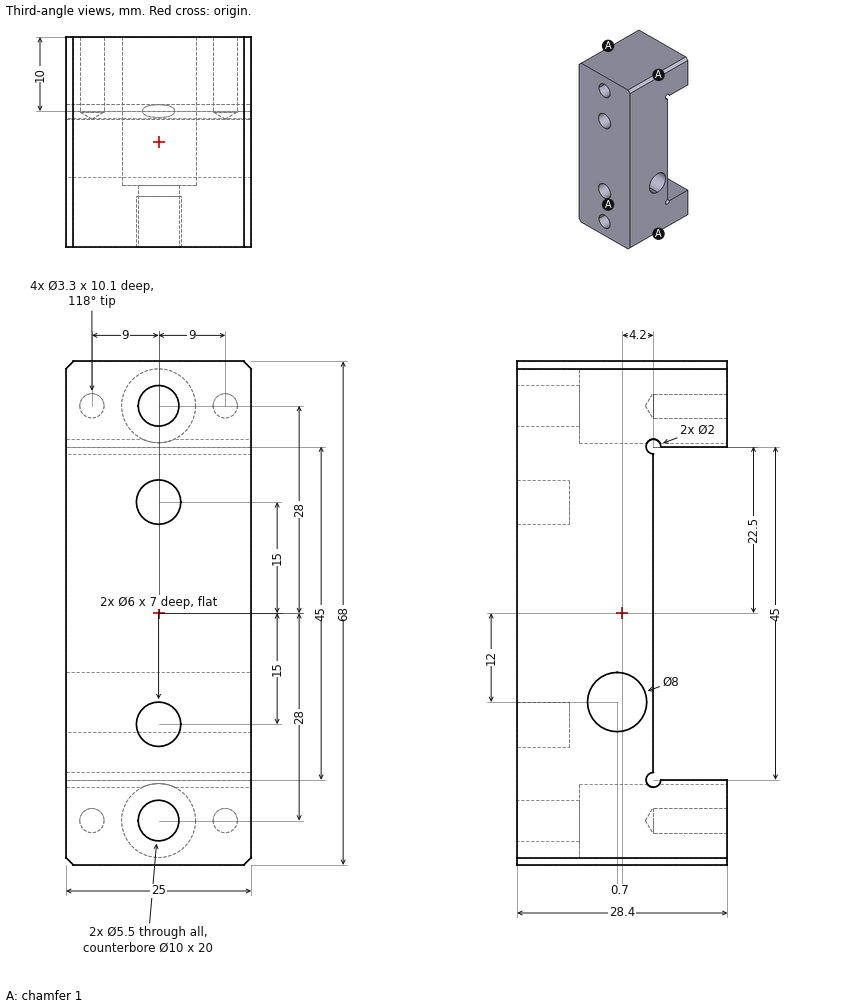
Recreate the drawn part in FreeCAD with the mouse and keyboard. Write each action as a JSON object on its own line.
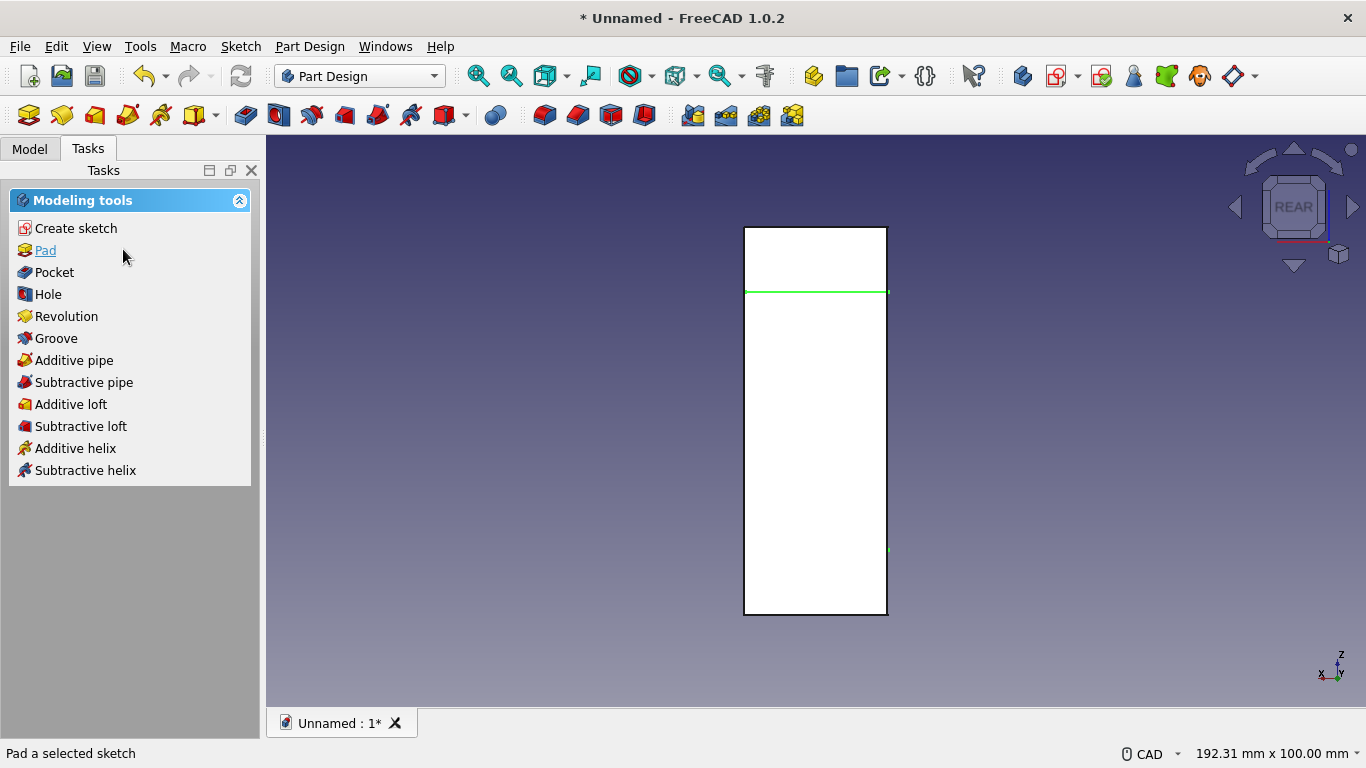
{"action": "left_click", "coordinate": [246, 116]}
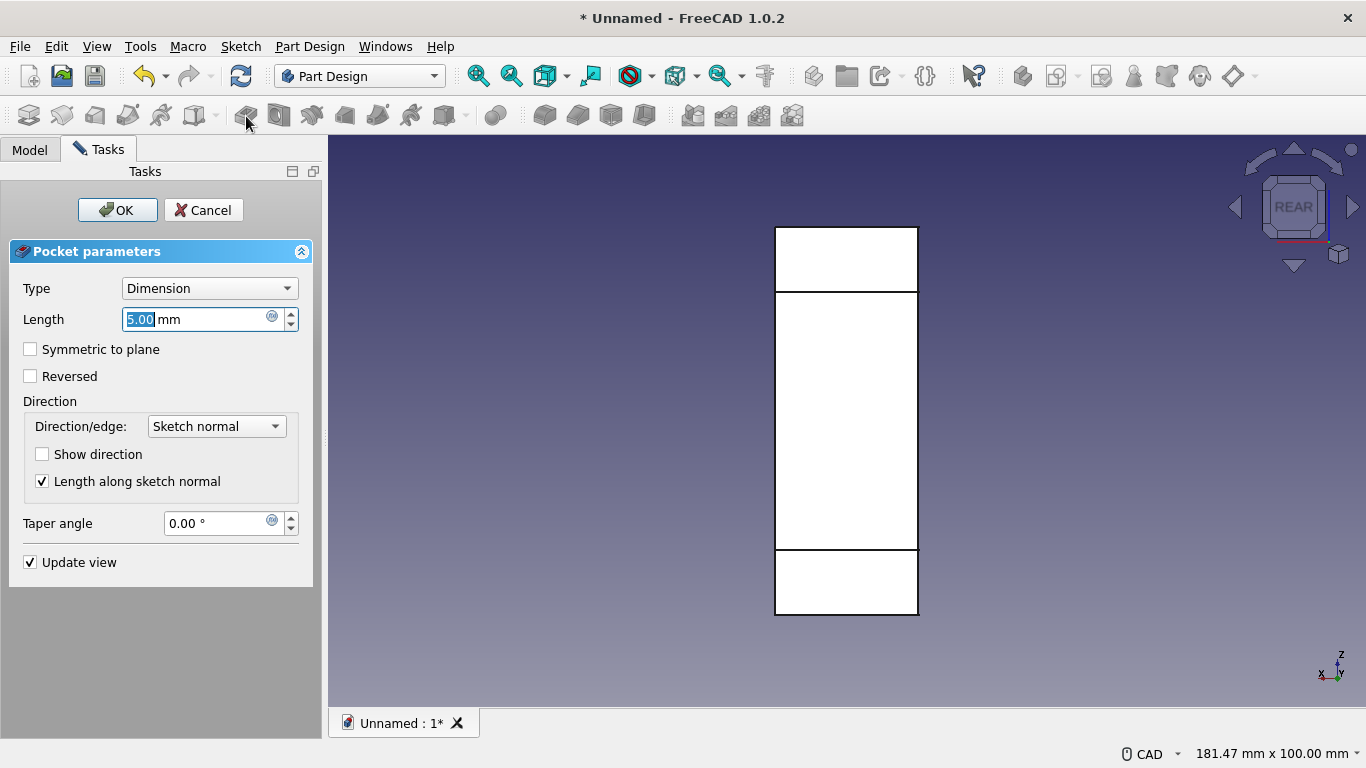
{"action": "left_click", "coordinate": [210, 288]}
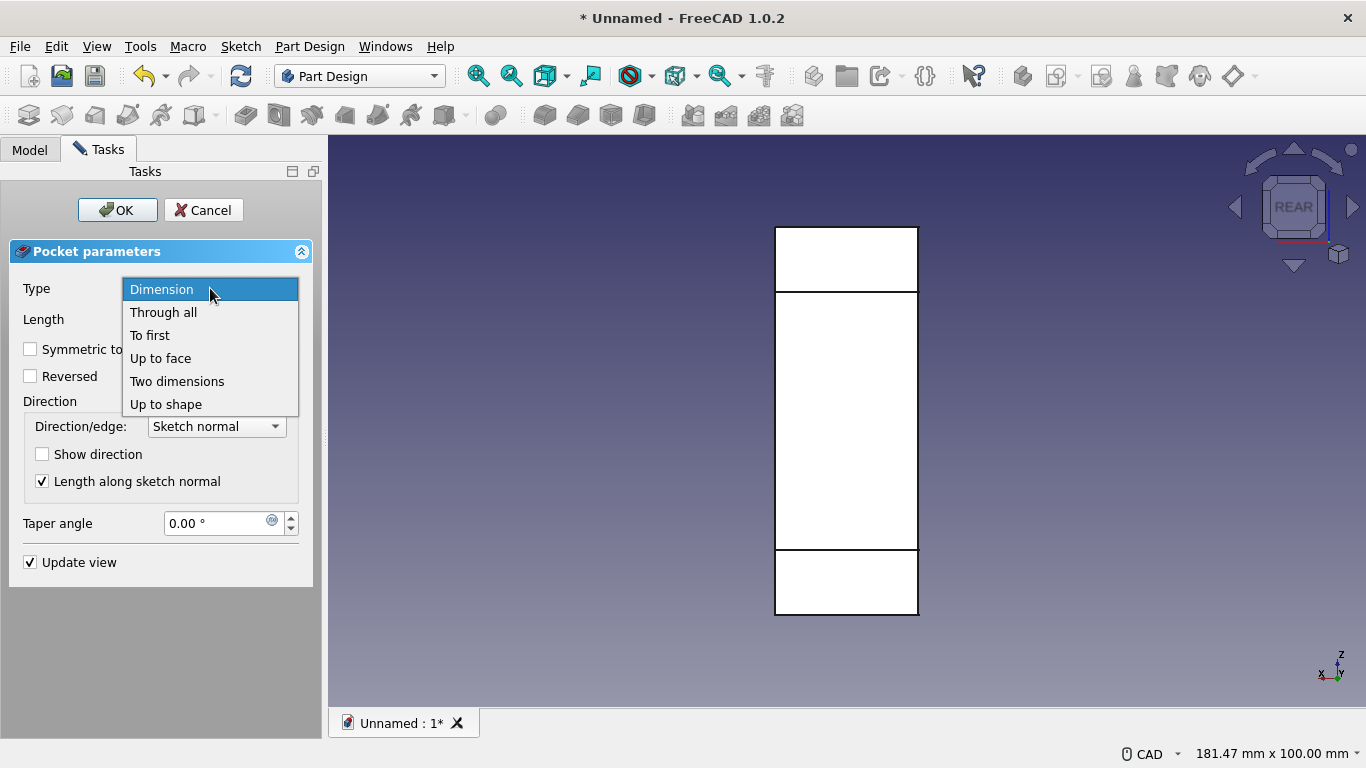
{"action": "left_click", "coordinate": [208, 382]}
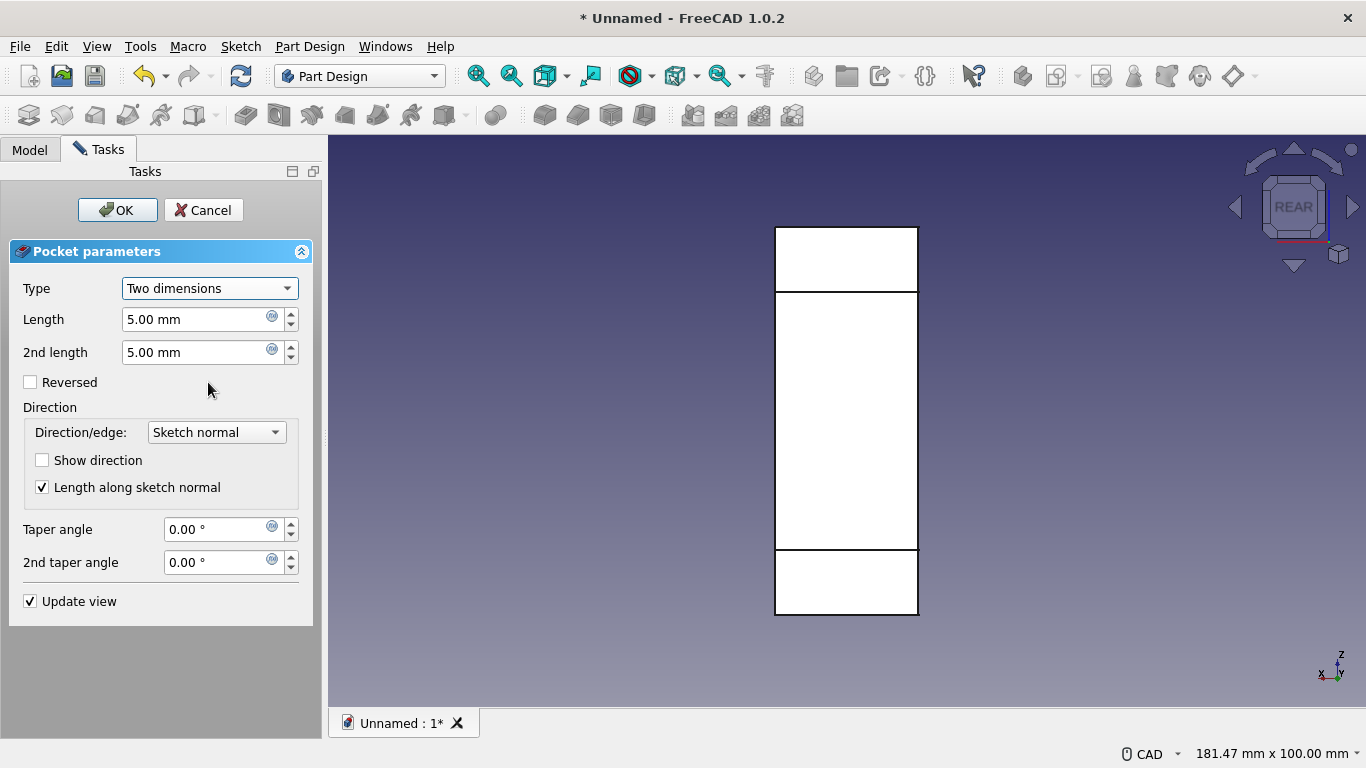
{"action": "triple_click", "coordinate": [204, 320]}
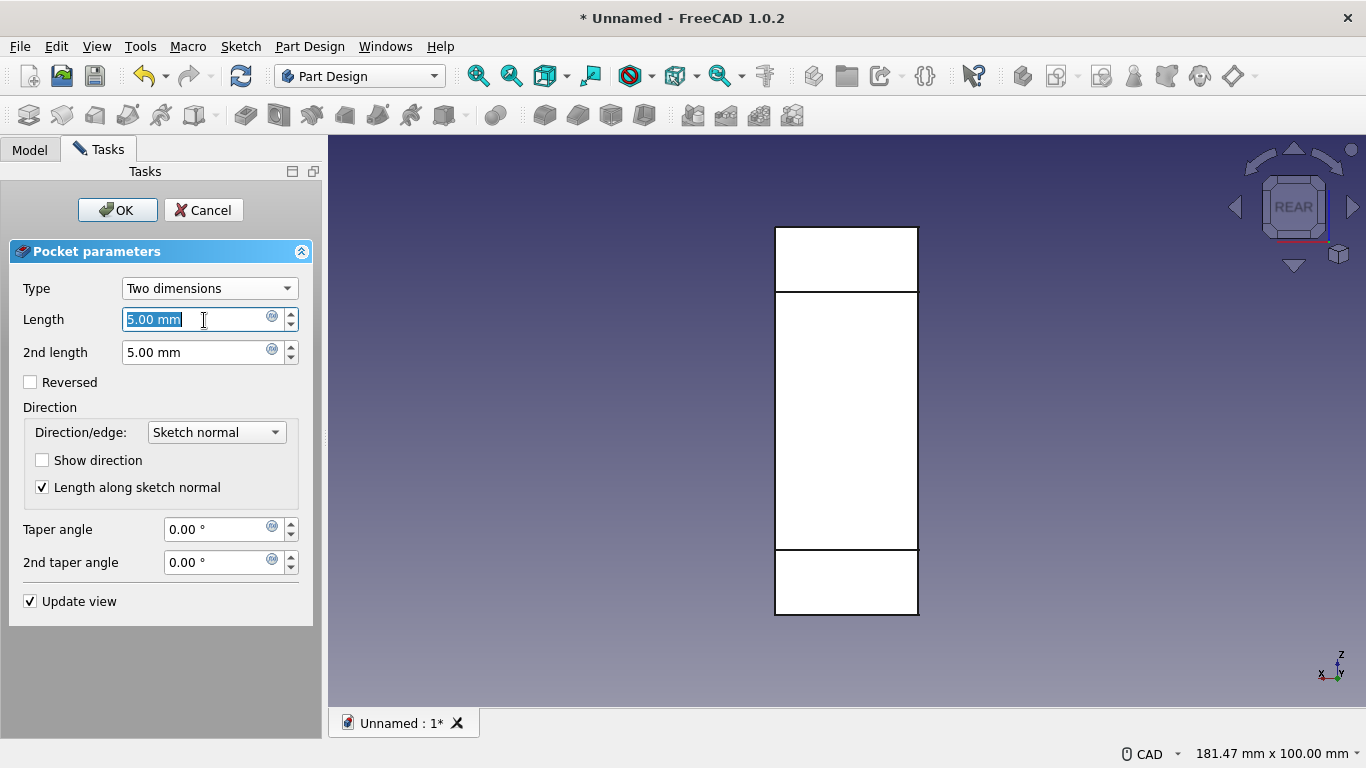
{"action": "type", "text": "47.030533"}
{"action": "key", "text": "Tab"}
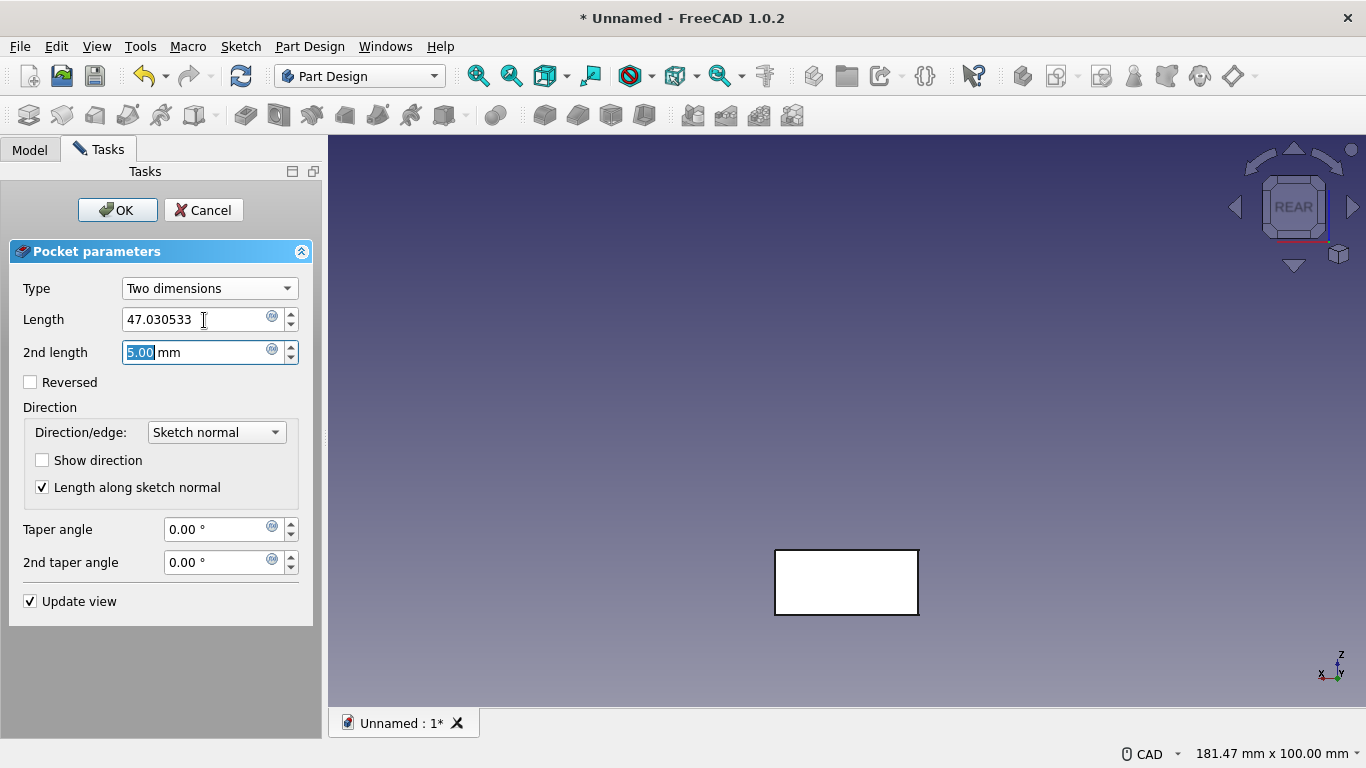
{"action": "type", "text": "10"}
{"action": "key", "text": "Tab"}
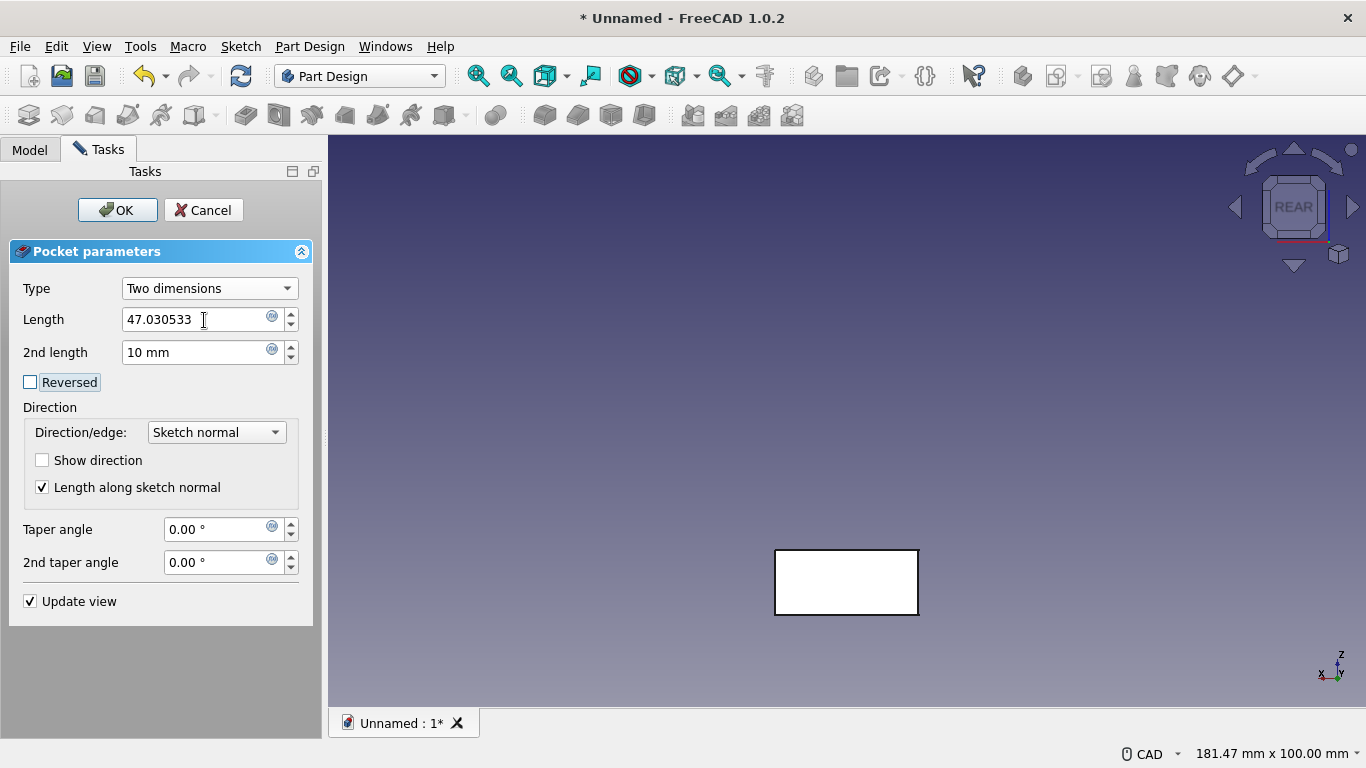
{"action": "left_click", "coordinate": [31, 382]}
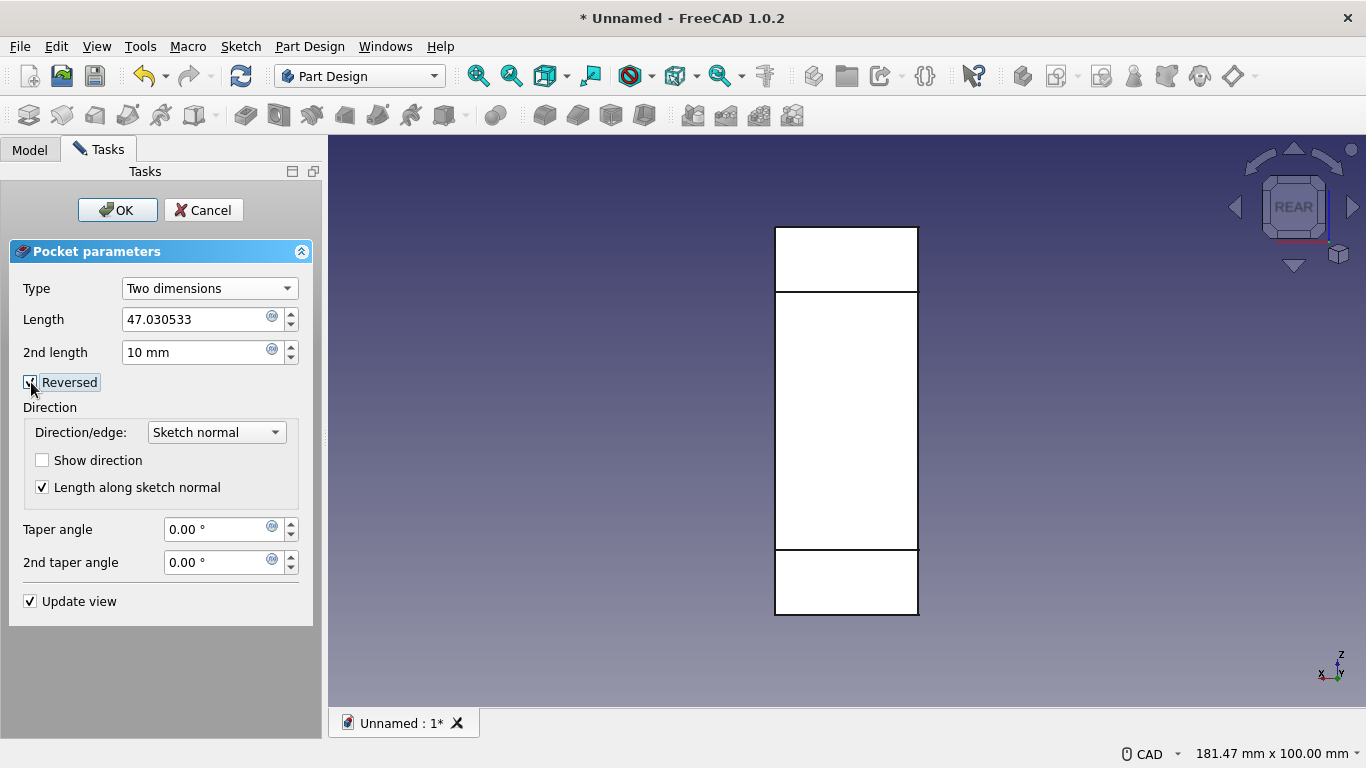
{"action": "left_click", "coordinate": [118, 210]}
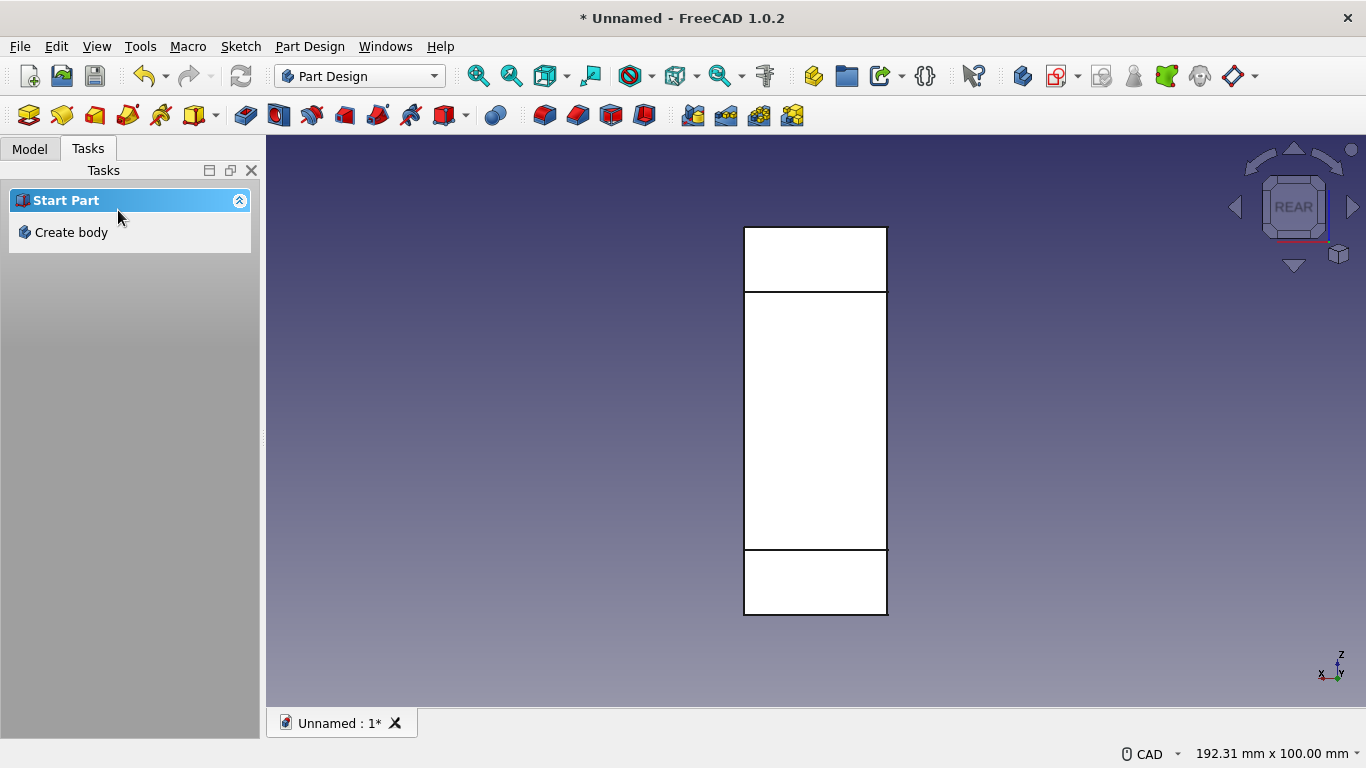
{"action": "key", "text": "0"}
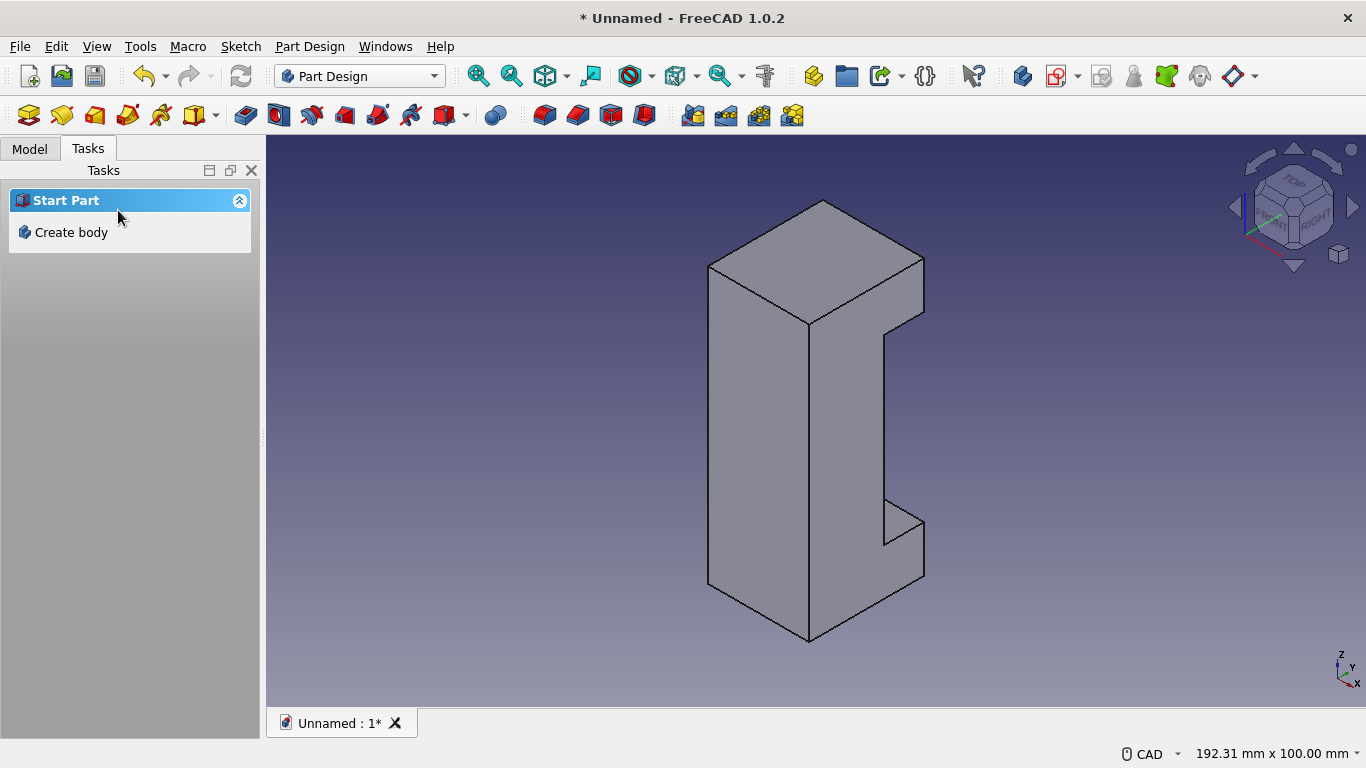
{"action": "left_click", "coordinate": [759, 362]}